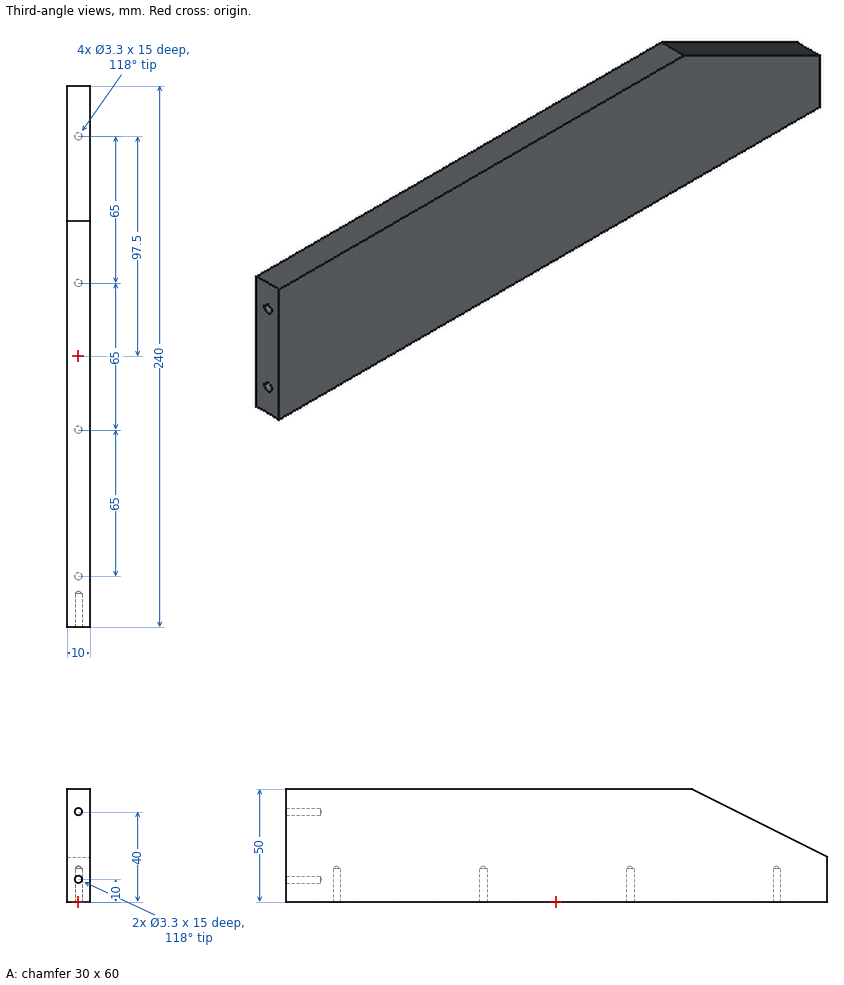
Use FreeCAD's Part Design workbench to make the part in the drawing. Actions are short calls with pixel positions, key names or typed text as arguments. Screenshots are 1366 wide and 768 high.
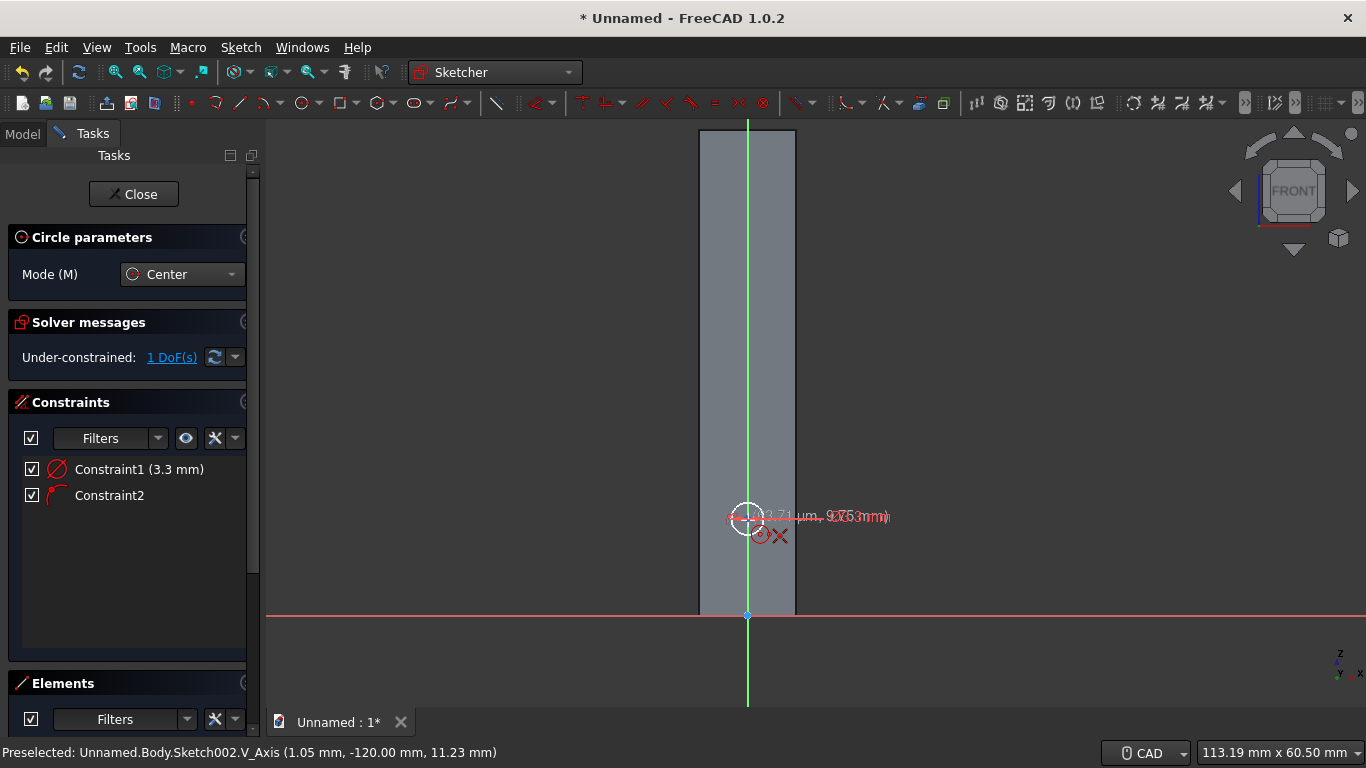
scroll(748, 227, up, 2)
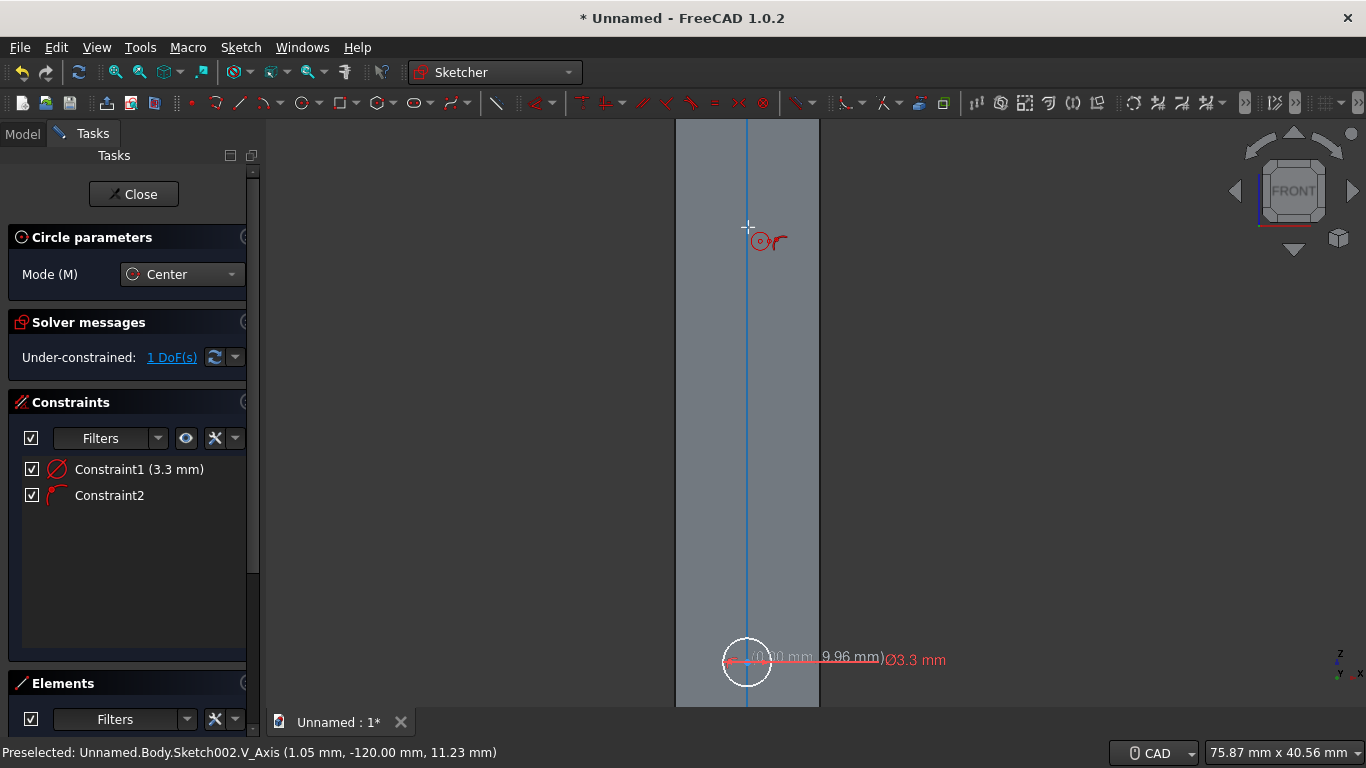
click(747, 227)
move(764, 210)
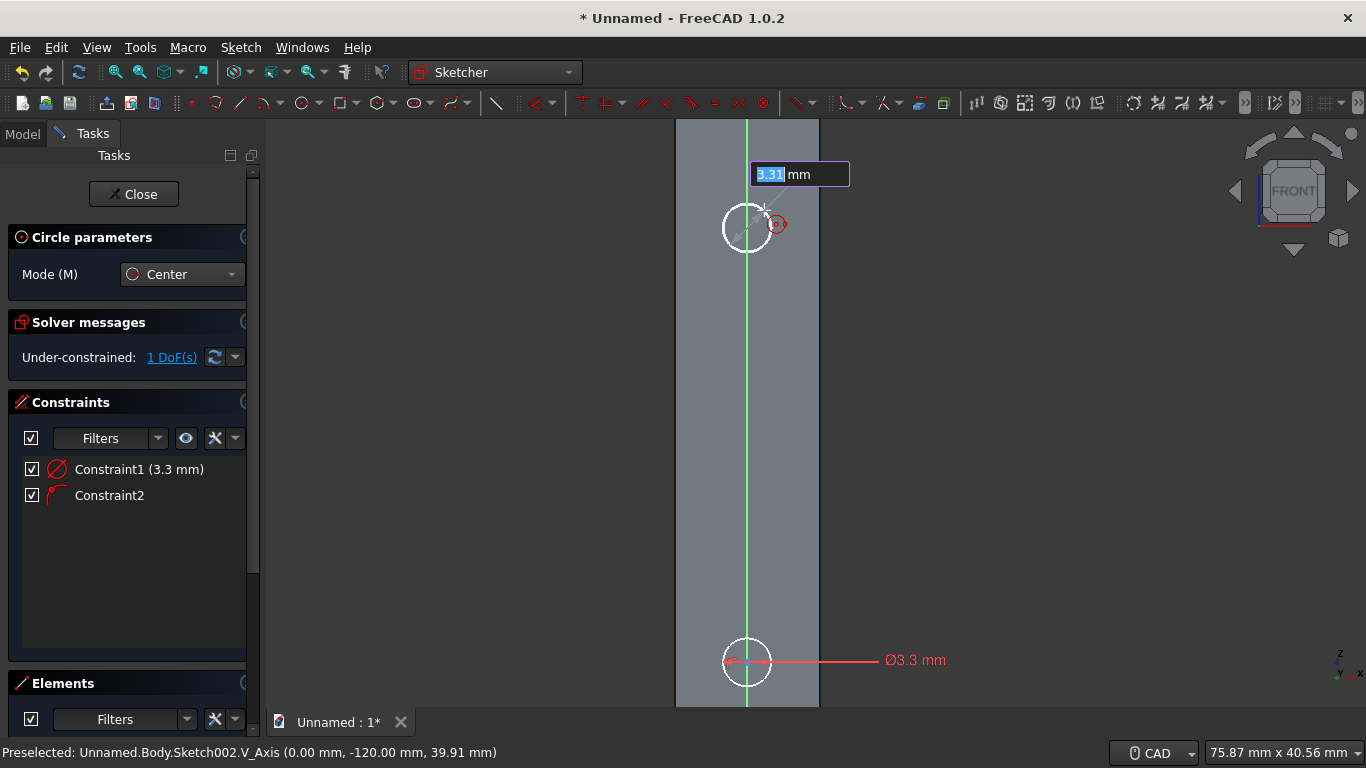
text(3.3)
key(Return)
key(Escape)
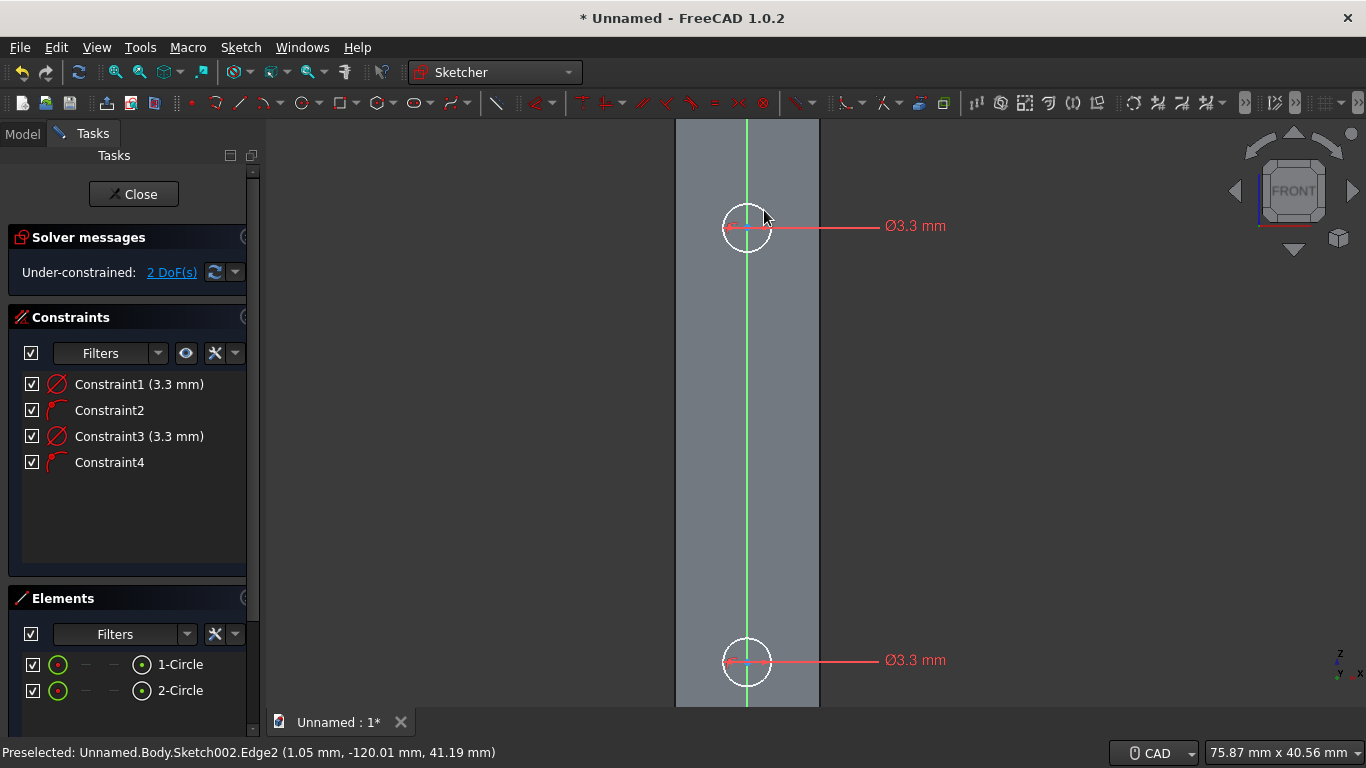
click(536, 104)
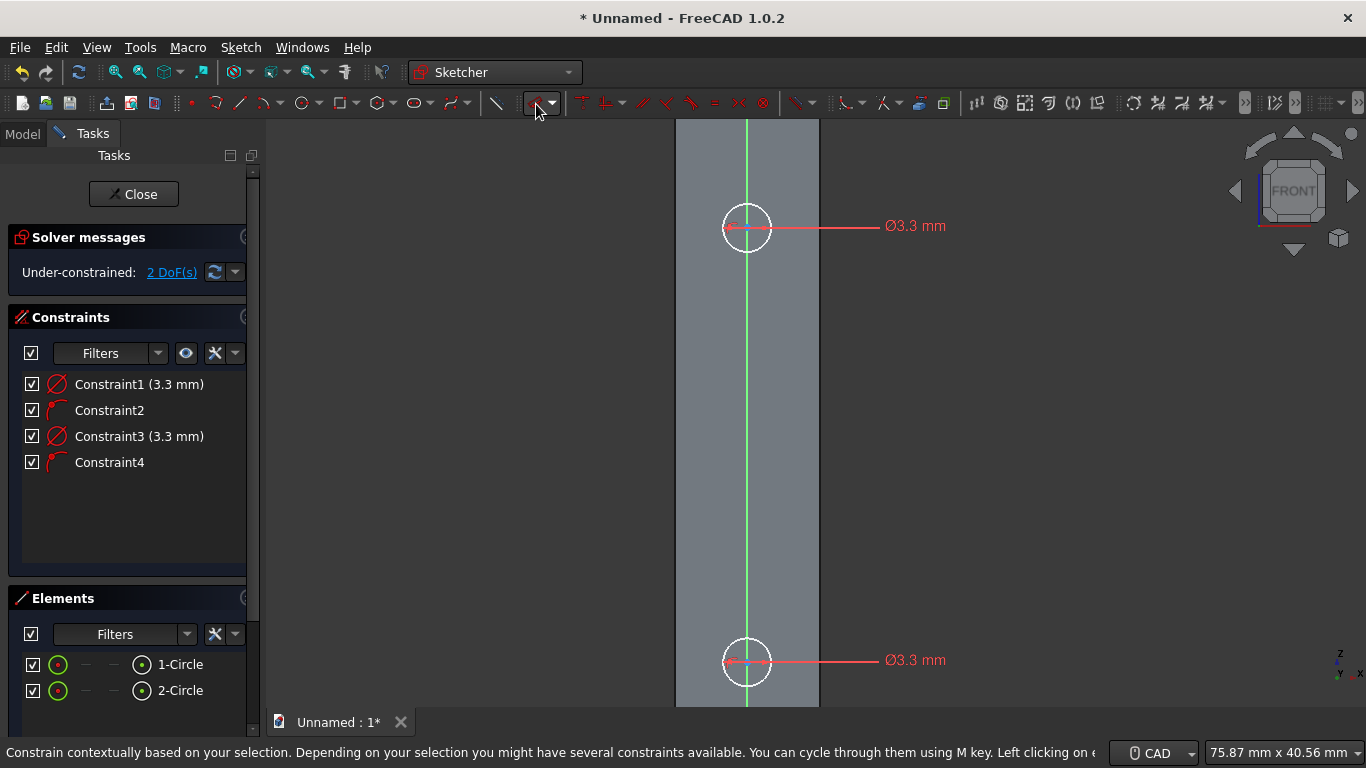
click(747, 662)
click(805, 671)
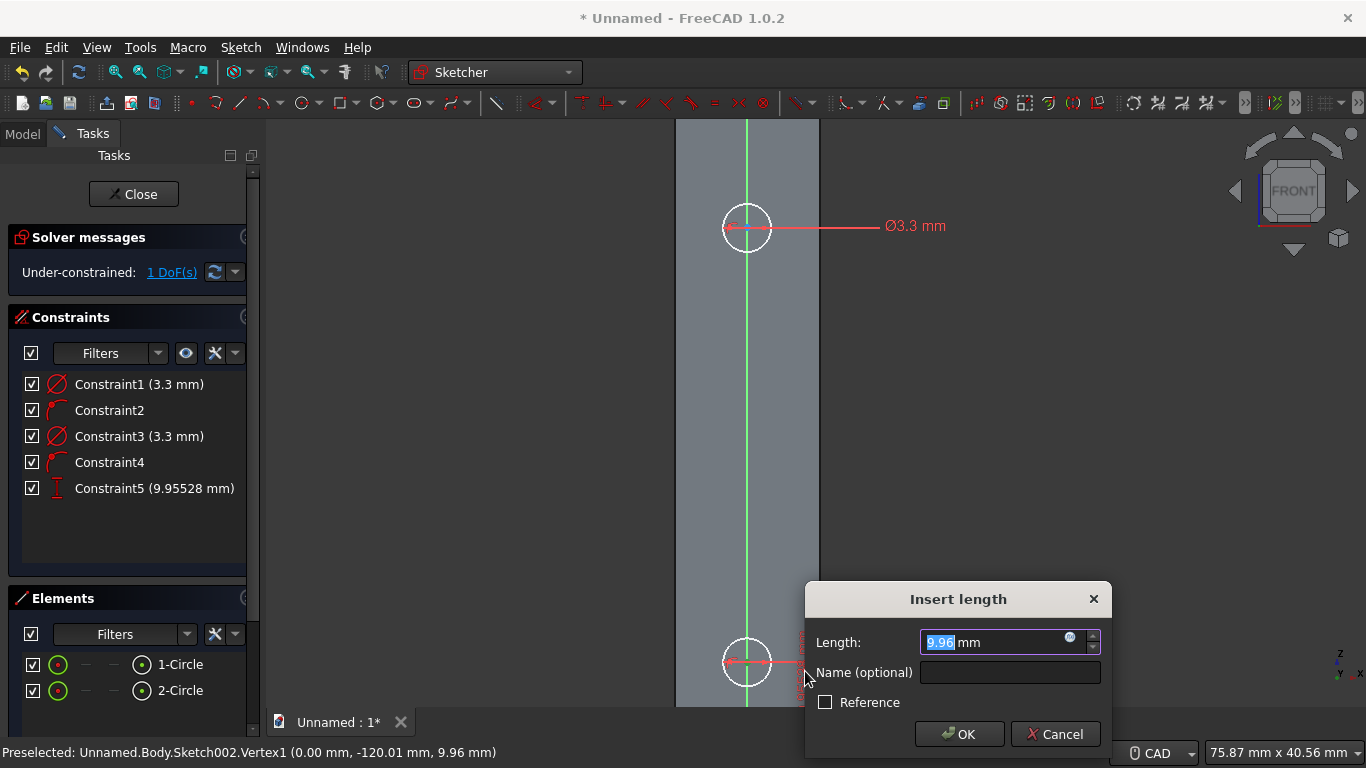
text(10)
key(Return)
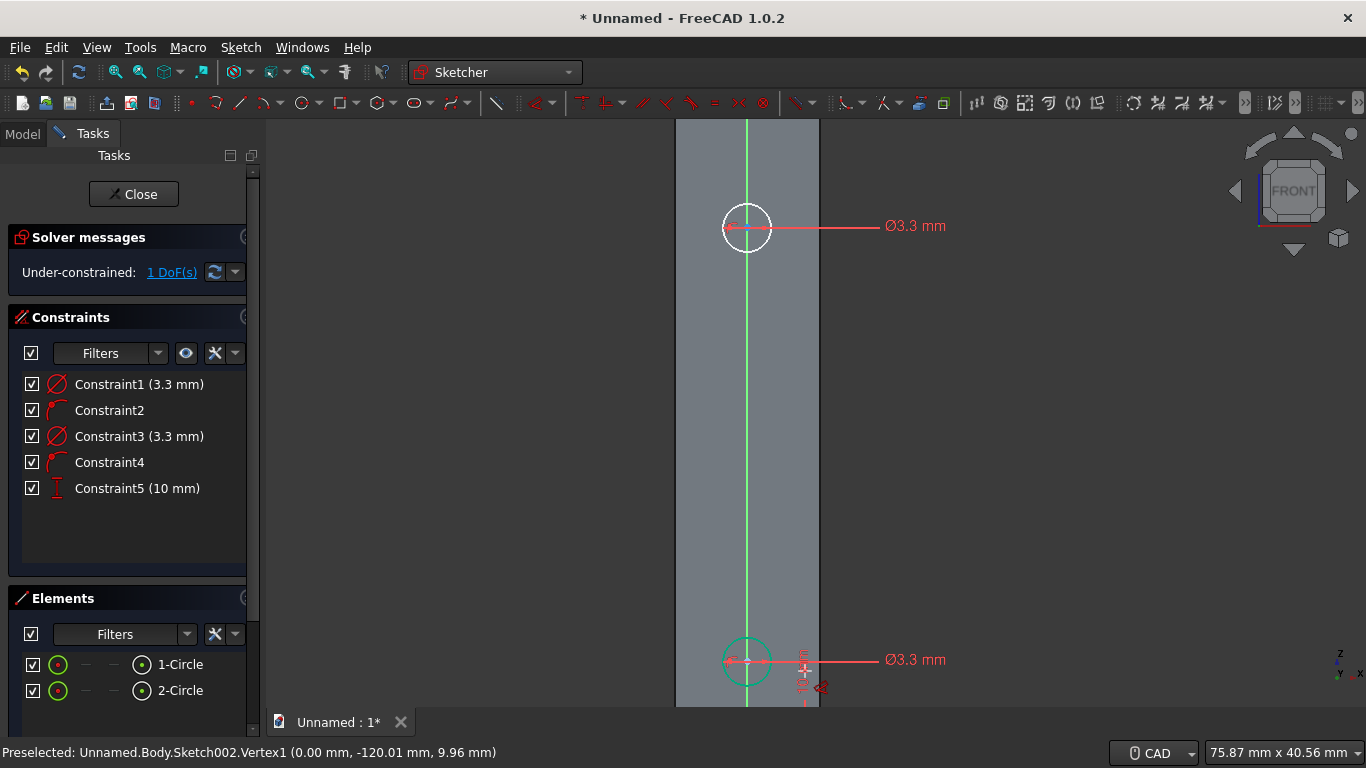
click(747, 228)
click(781, 453)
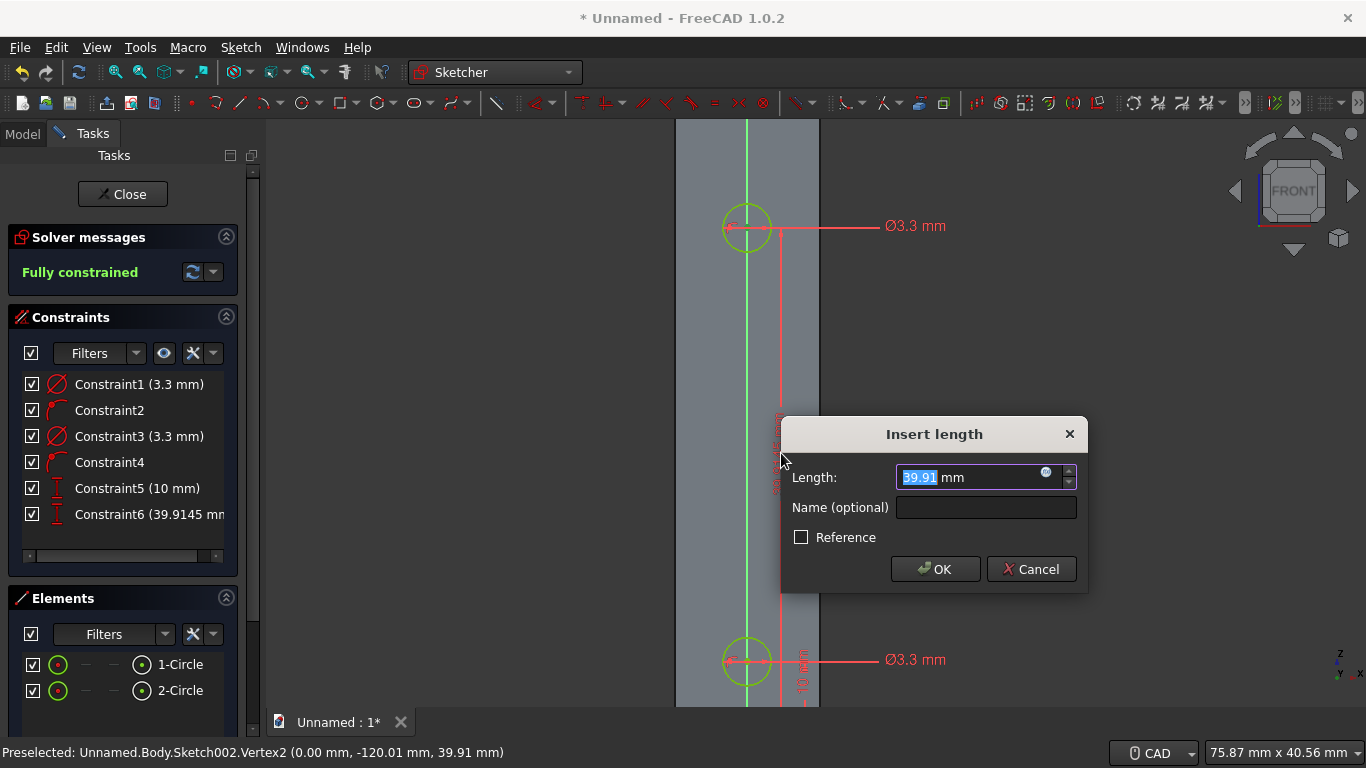
text(40)
key(Return)
key(Escape)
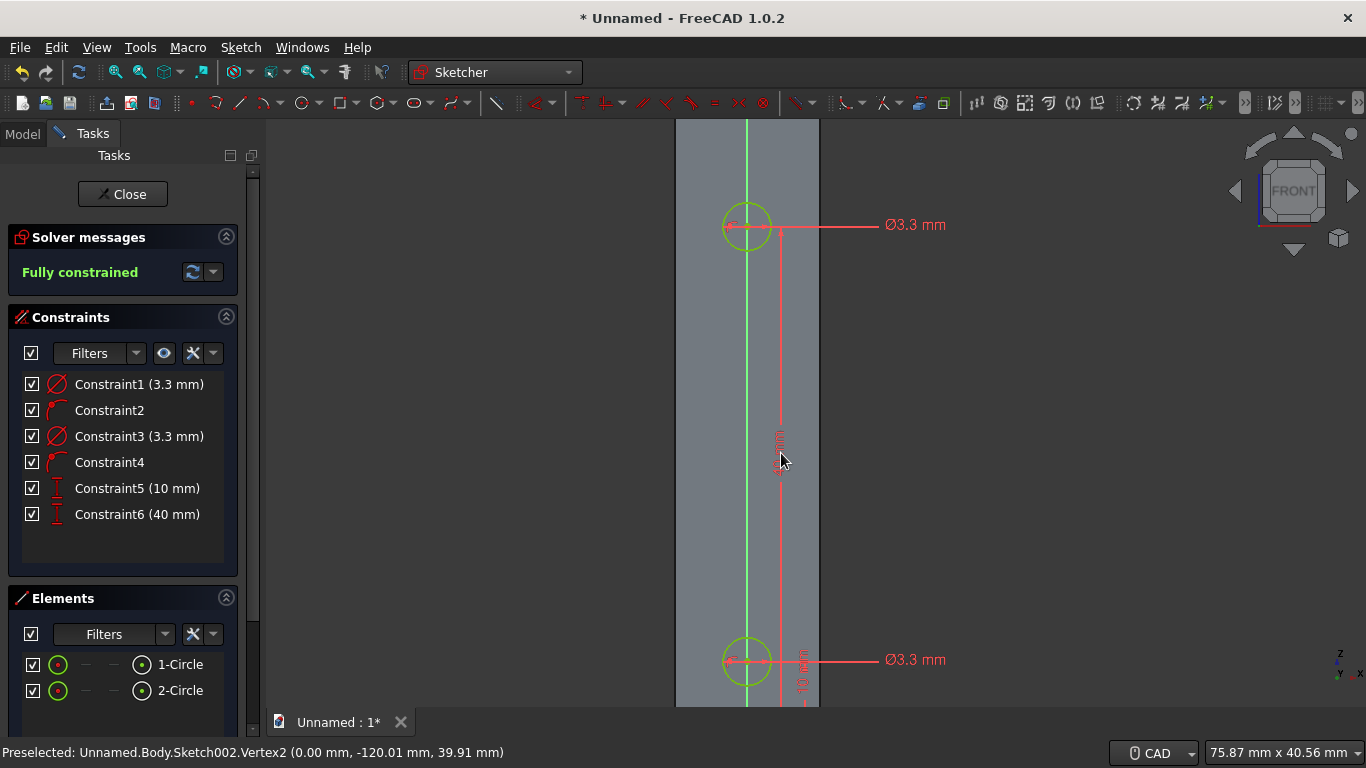
click(123, 194)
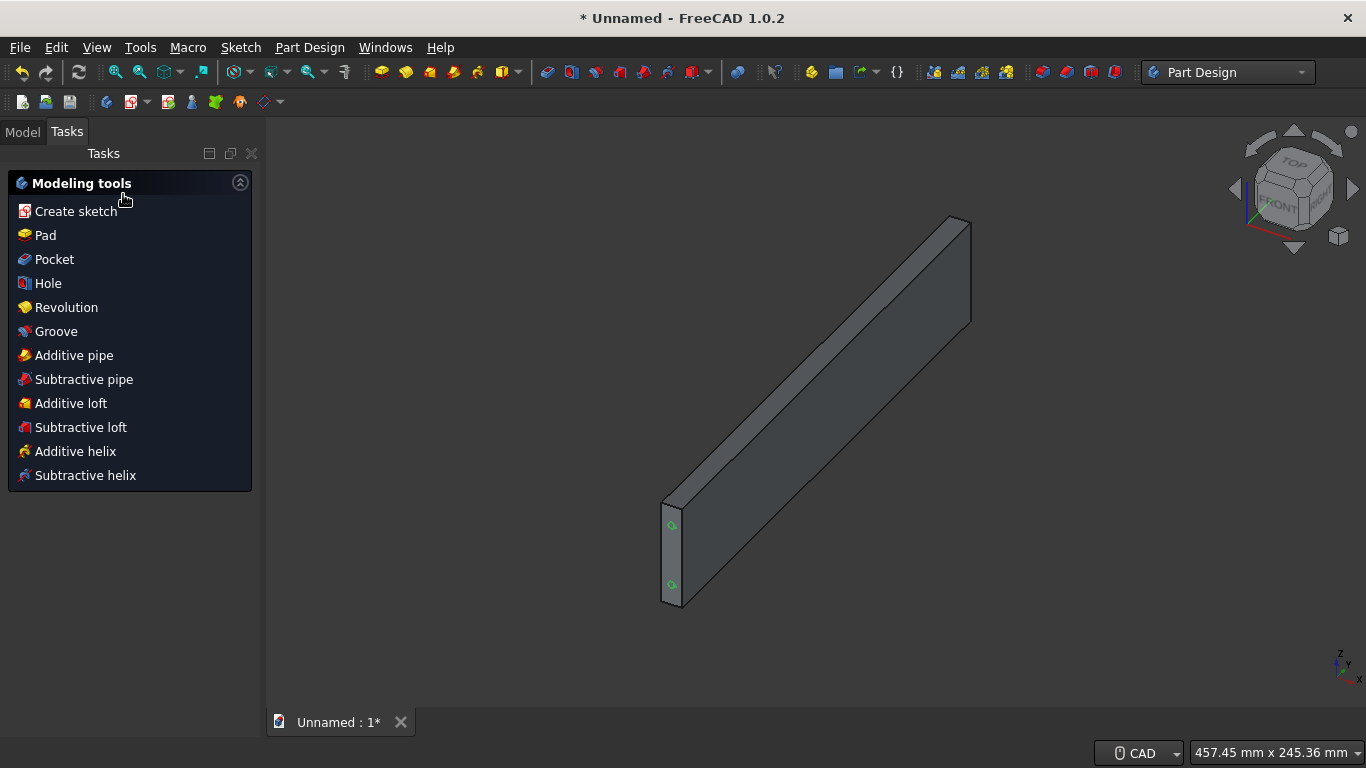
click(572, 72)